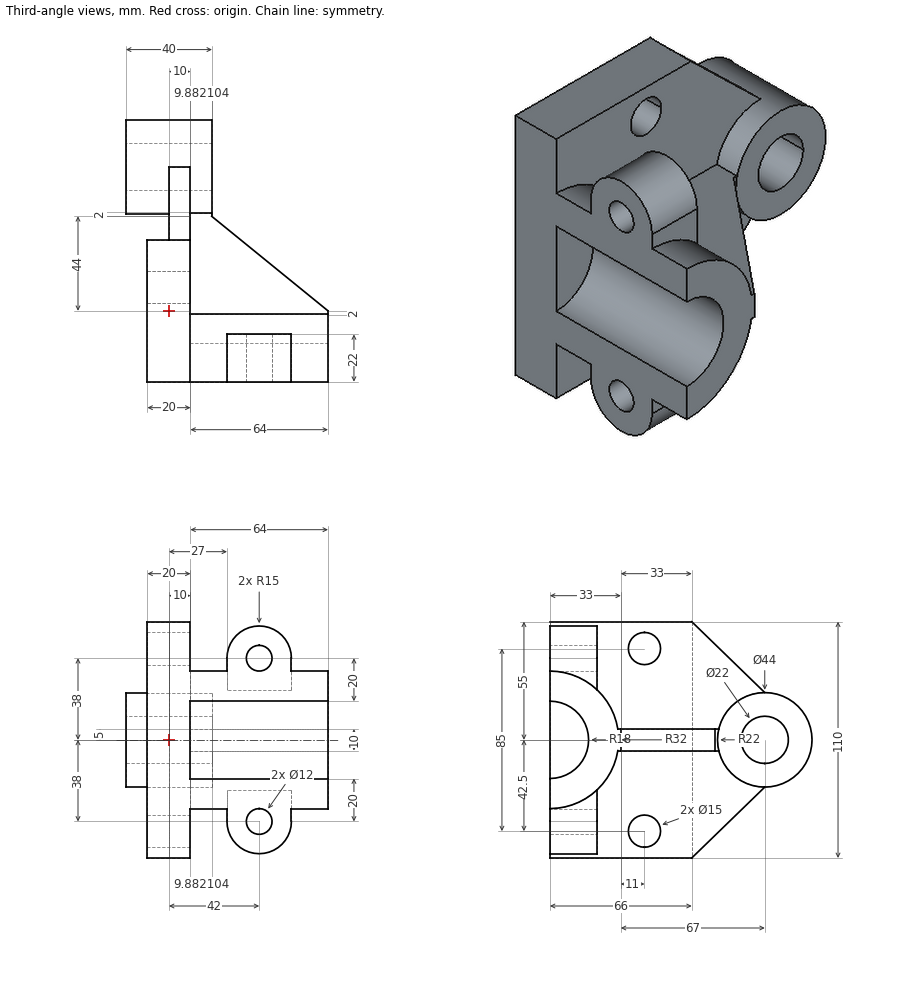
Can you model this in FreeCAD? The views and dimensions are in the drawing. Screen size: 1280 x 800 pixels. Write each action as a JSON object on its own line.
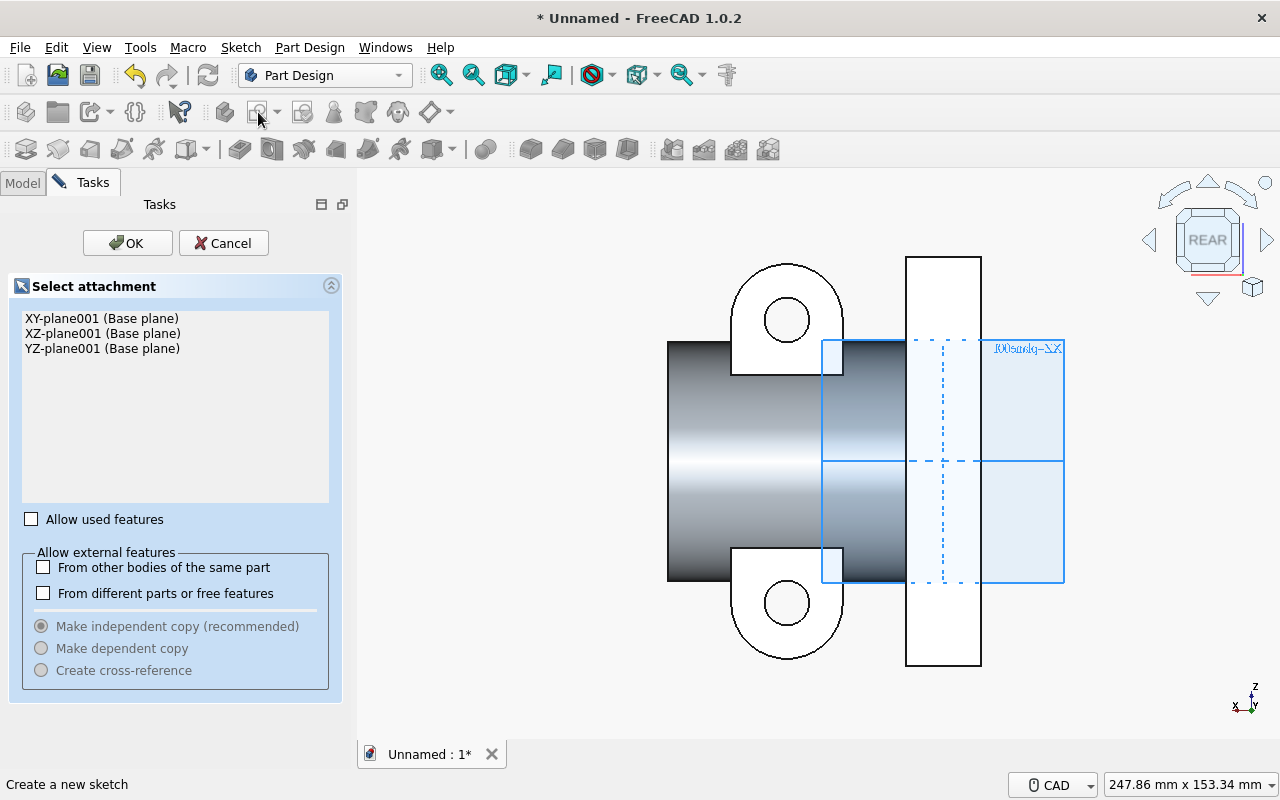
{"action": "left_click", "coordinate": [82, 348]}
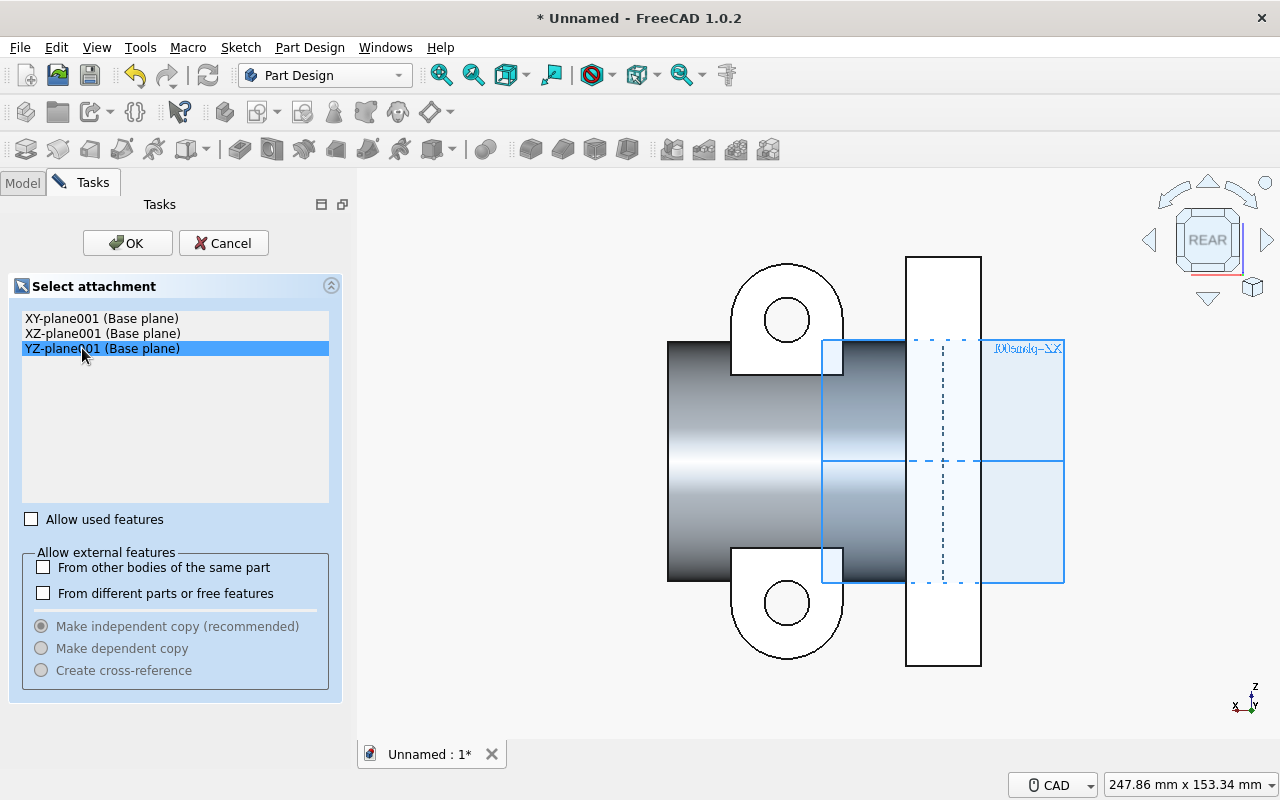
{"action": "left_click", "coordinate": [128, 243]}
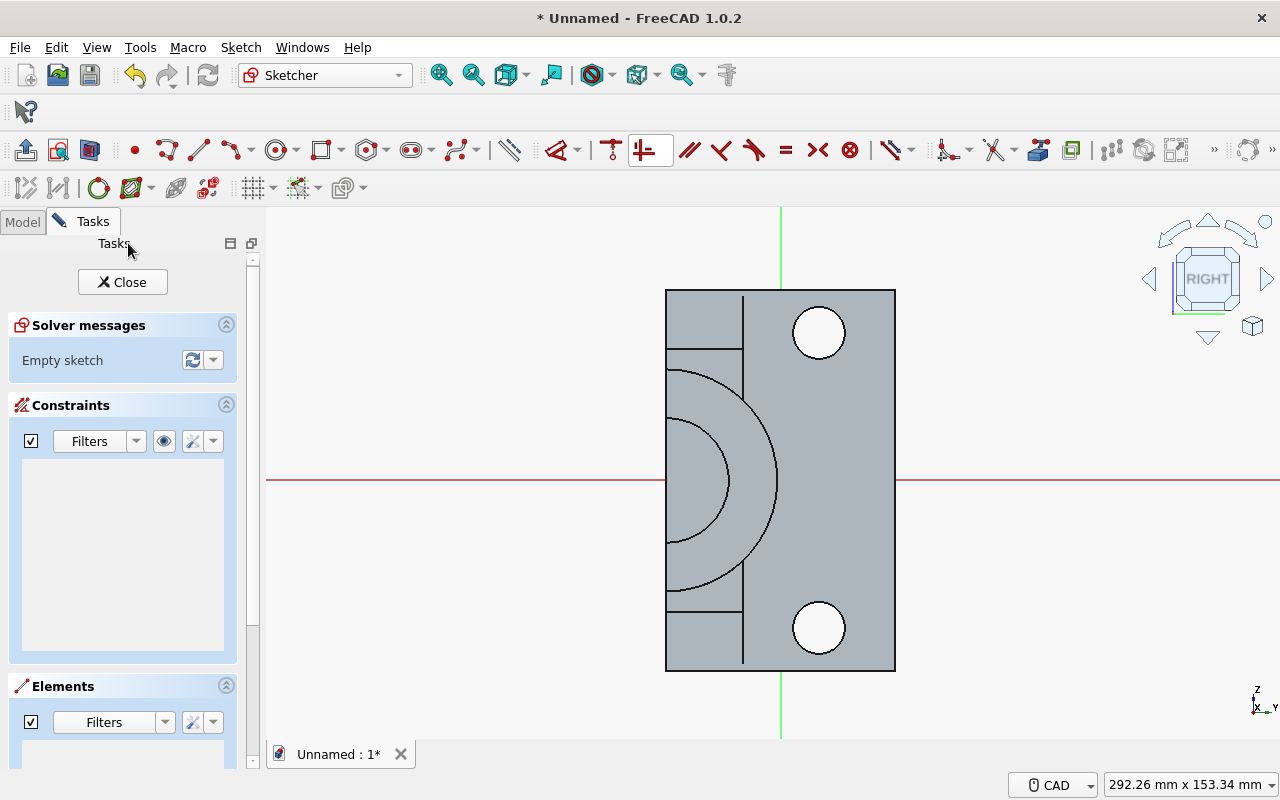
{"action": "scroll", "coordinate": [1115, 489], "scroll_direction": "up", "scroll_amount": 3}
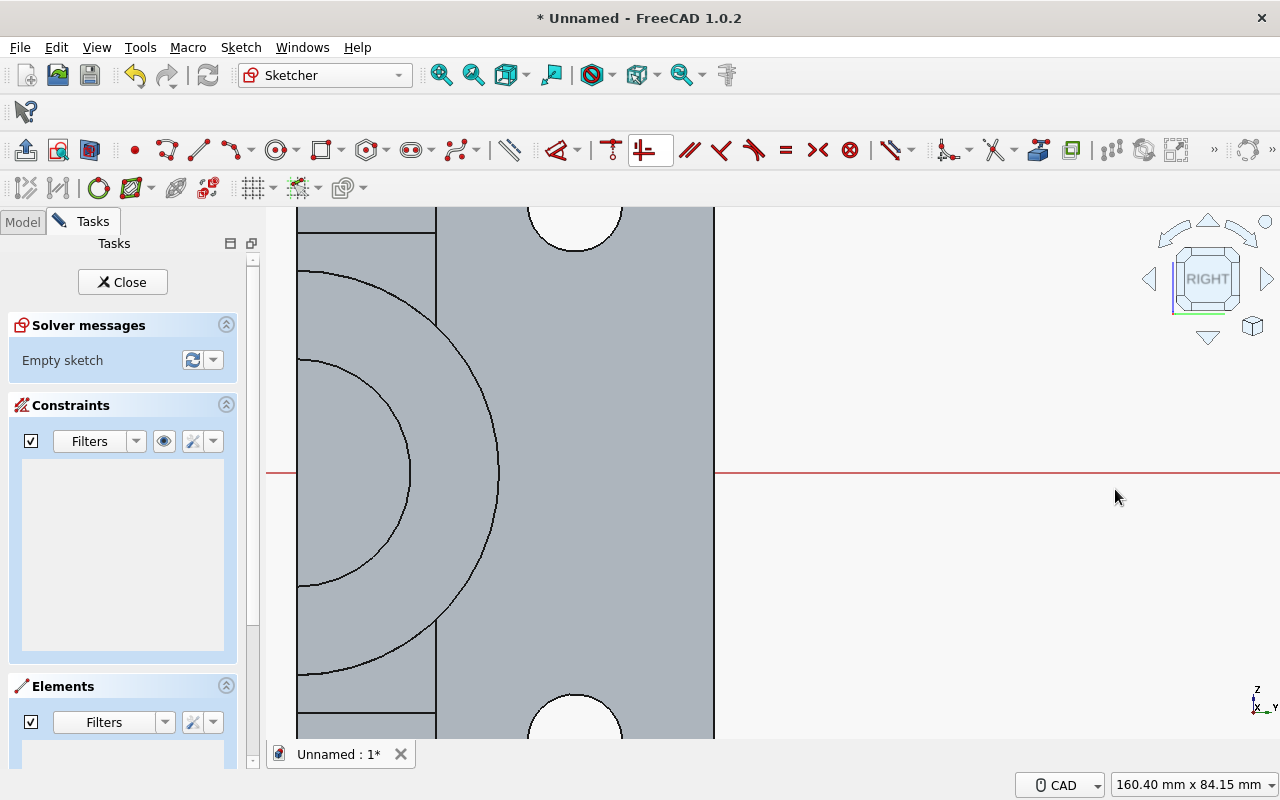
{"action": "left_click", "coordinate": [276, 150]}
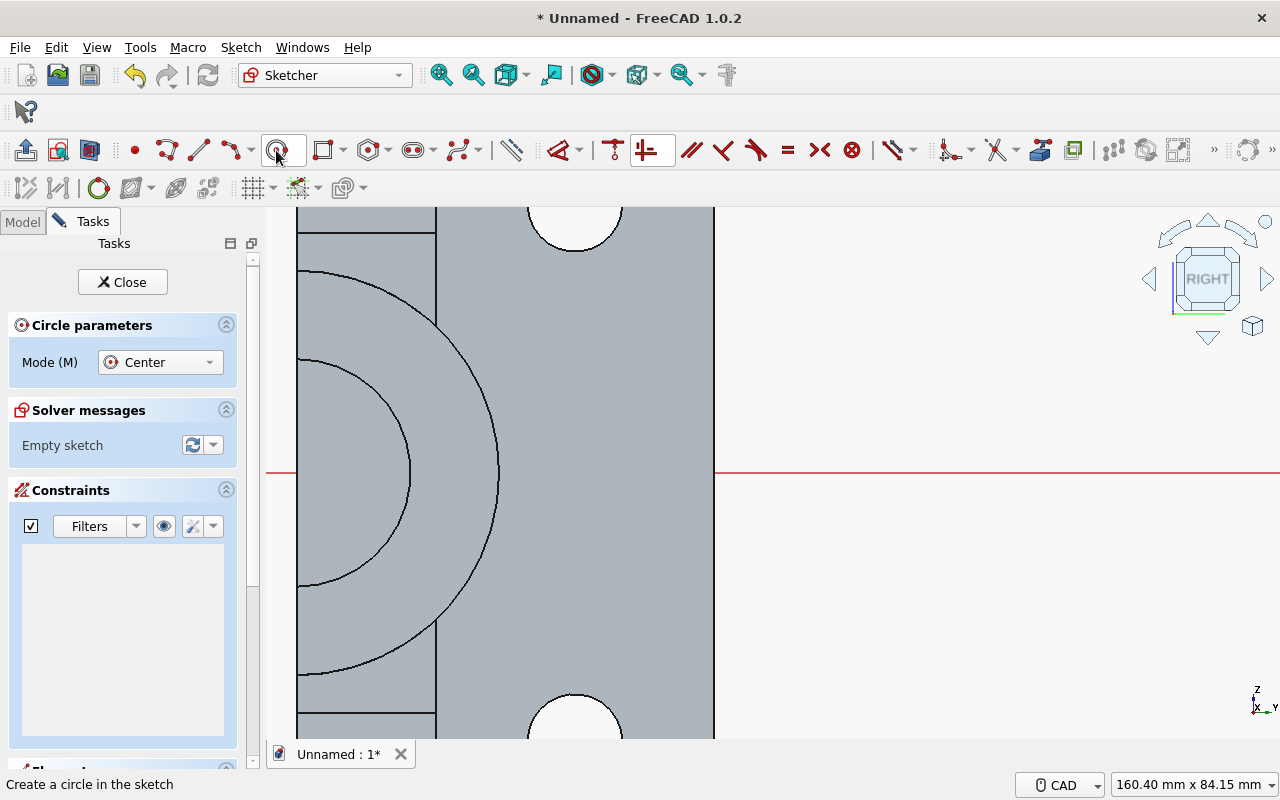
{"action": "left_click", "coordinate": [929, 473]}
{"action": "left_click", "coordinate": [1027, 375]}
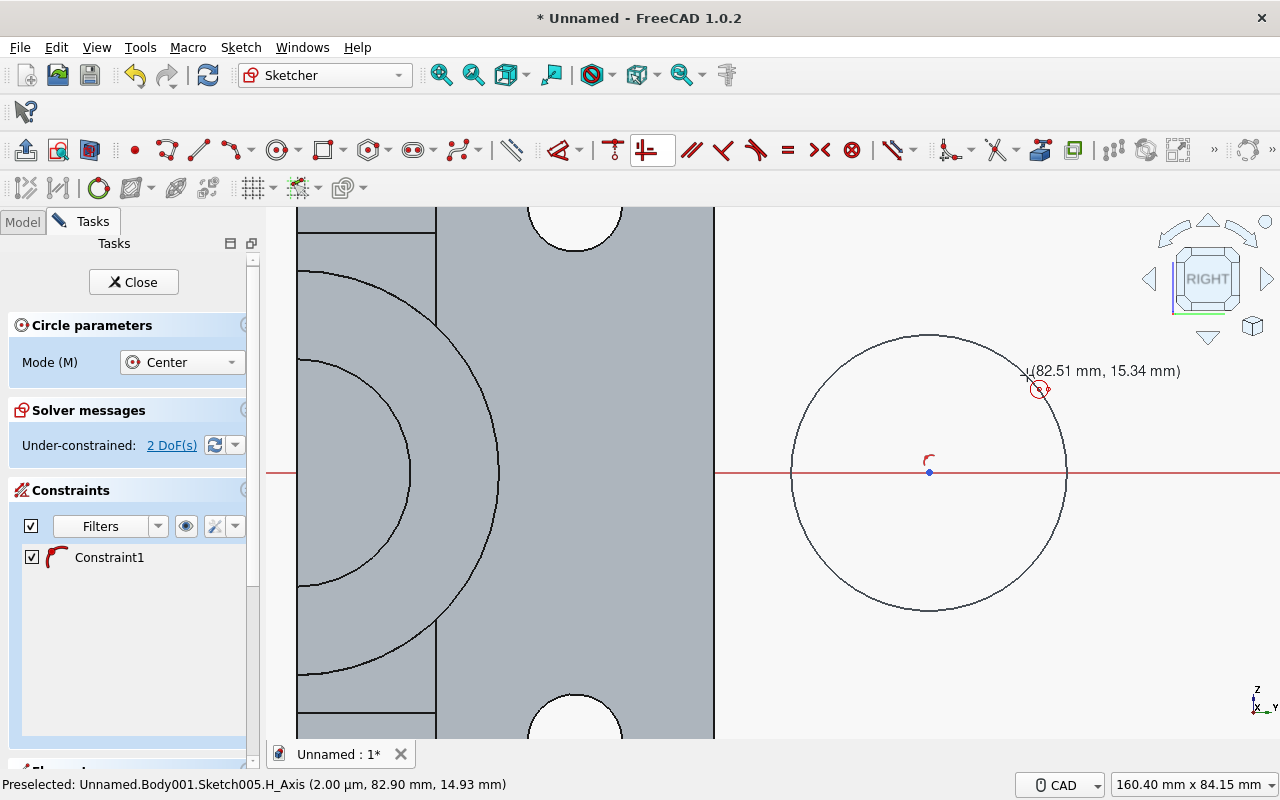
{"action": "left_click", "coordinate": [929, 473]}
{"action": "left_click", "coordinate": [978, 424]}
{"action": "key", "text": "Escape"}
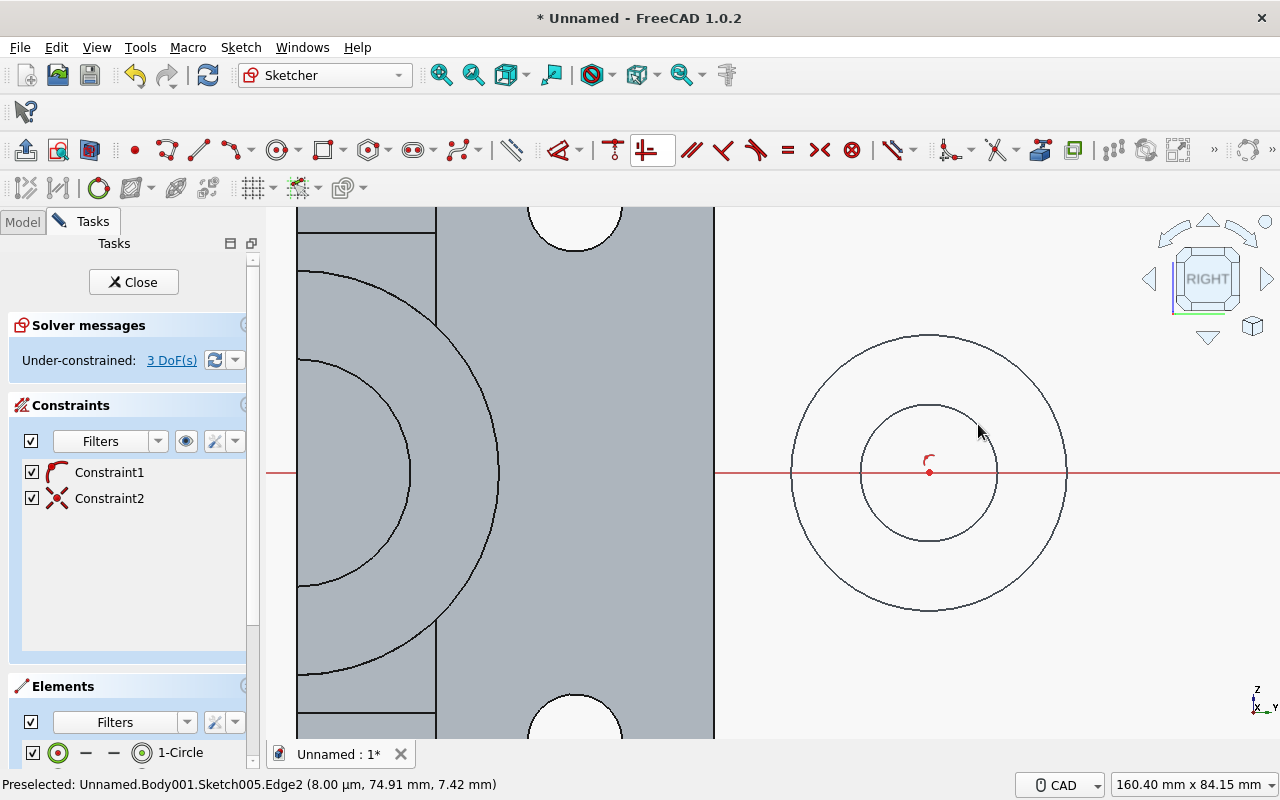
{"action": "left_click", "coordinate": [558, 150]}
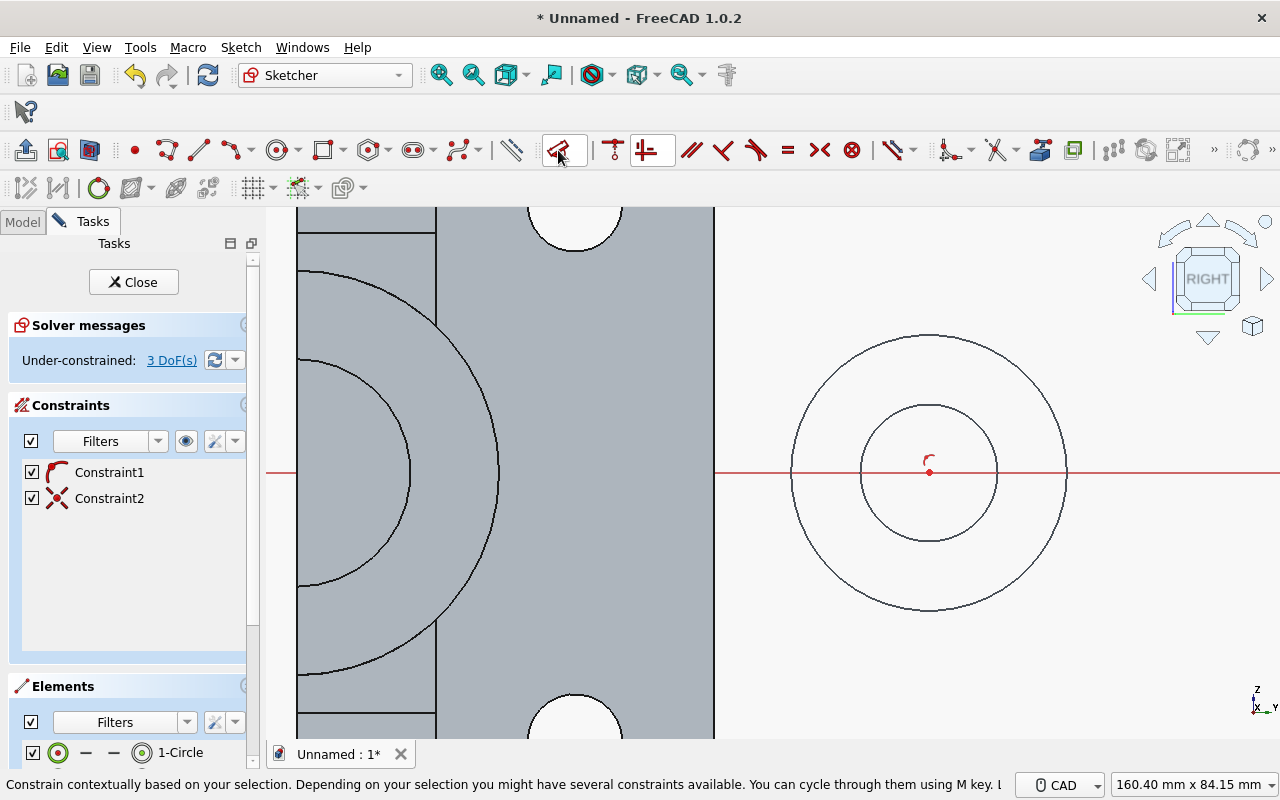
{"action": "left_click", "coordinate": [1026, 375]}
{"action": "left_click", "coordinate": [1049, 352]}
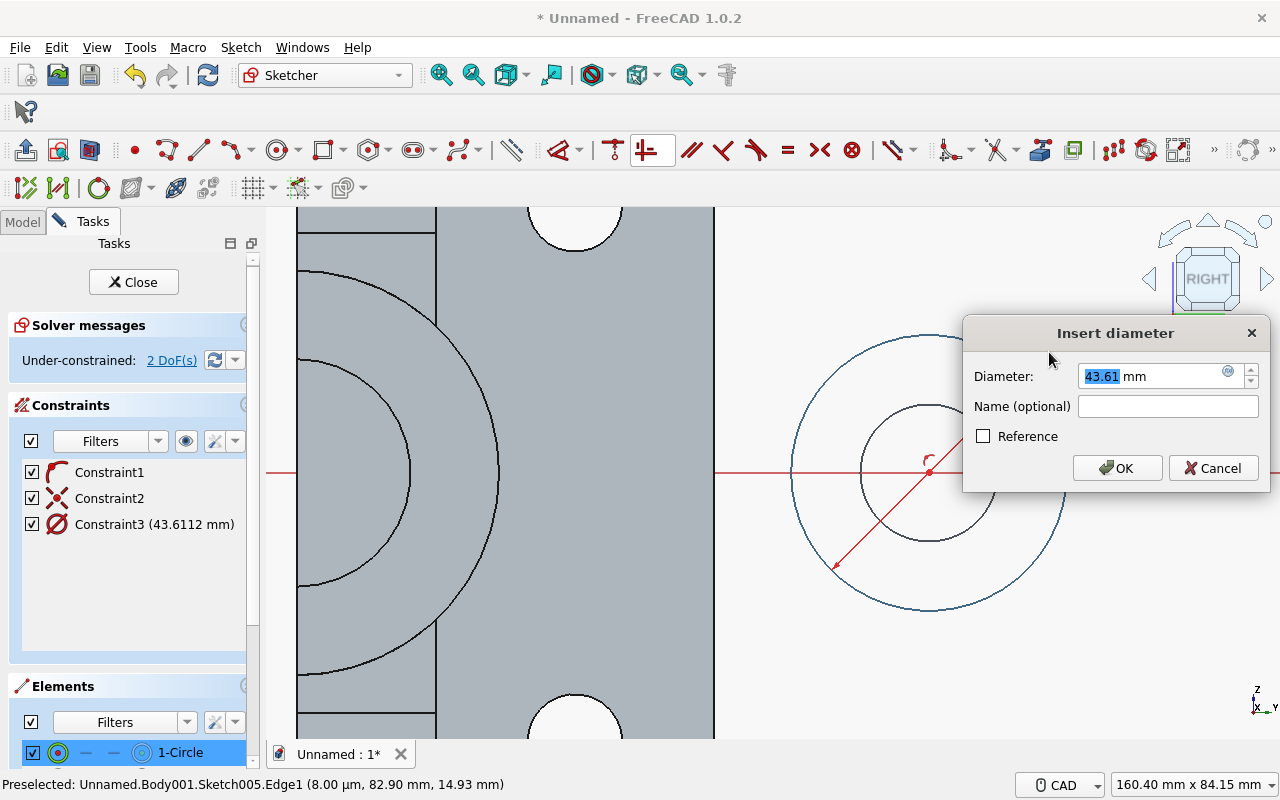
{"action": "type", "text": "44"}
{"action": "key", "text": "Return"}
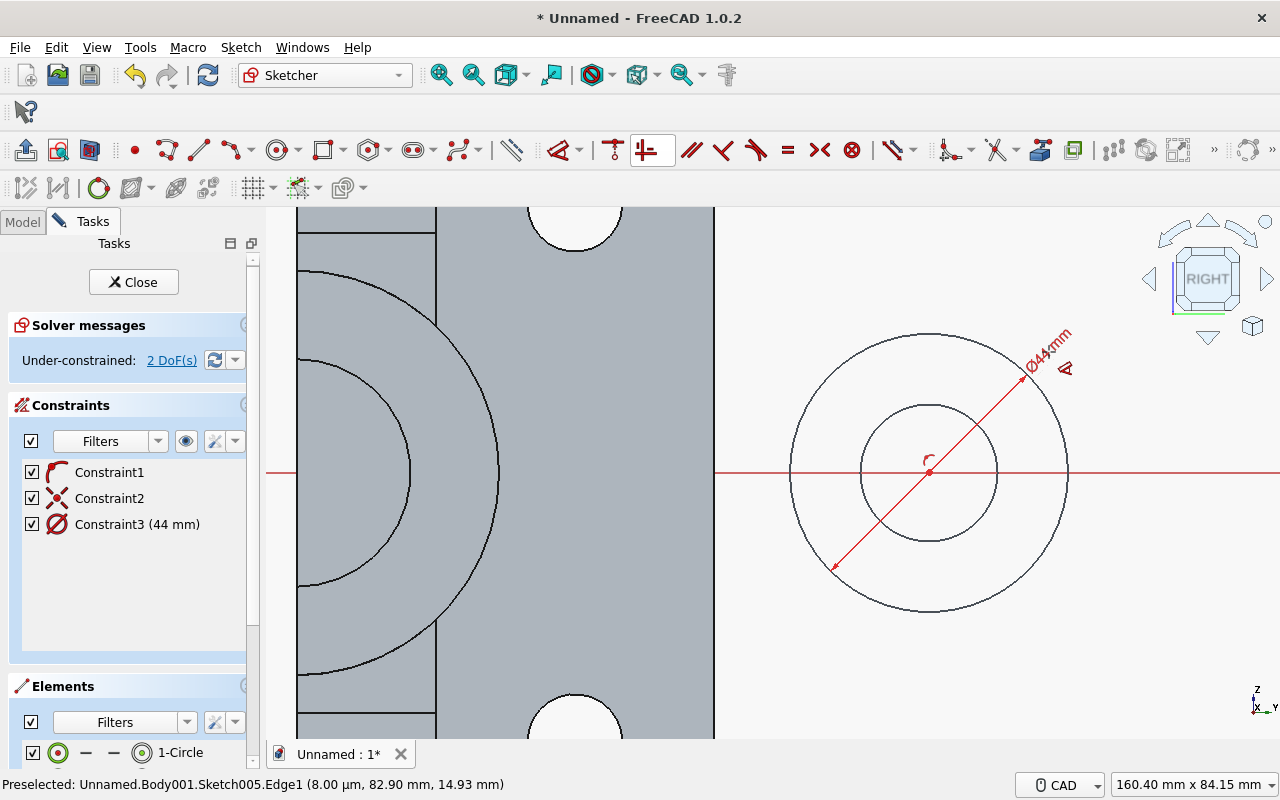
{"action": "left_click", "coordinate": [977, 424]}
{"action": "left_click", "coordinate": [999, 401]}